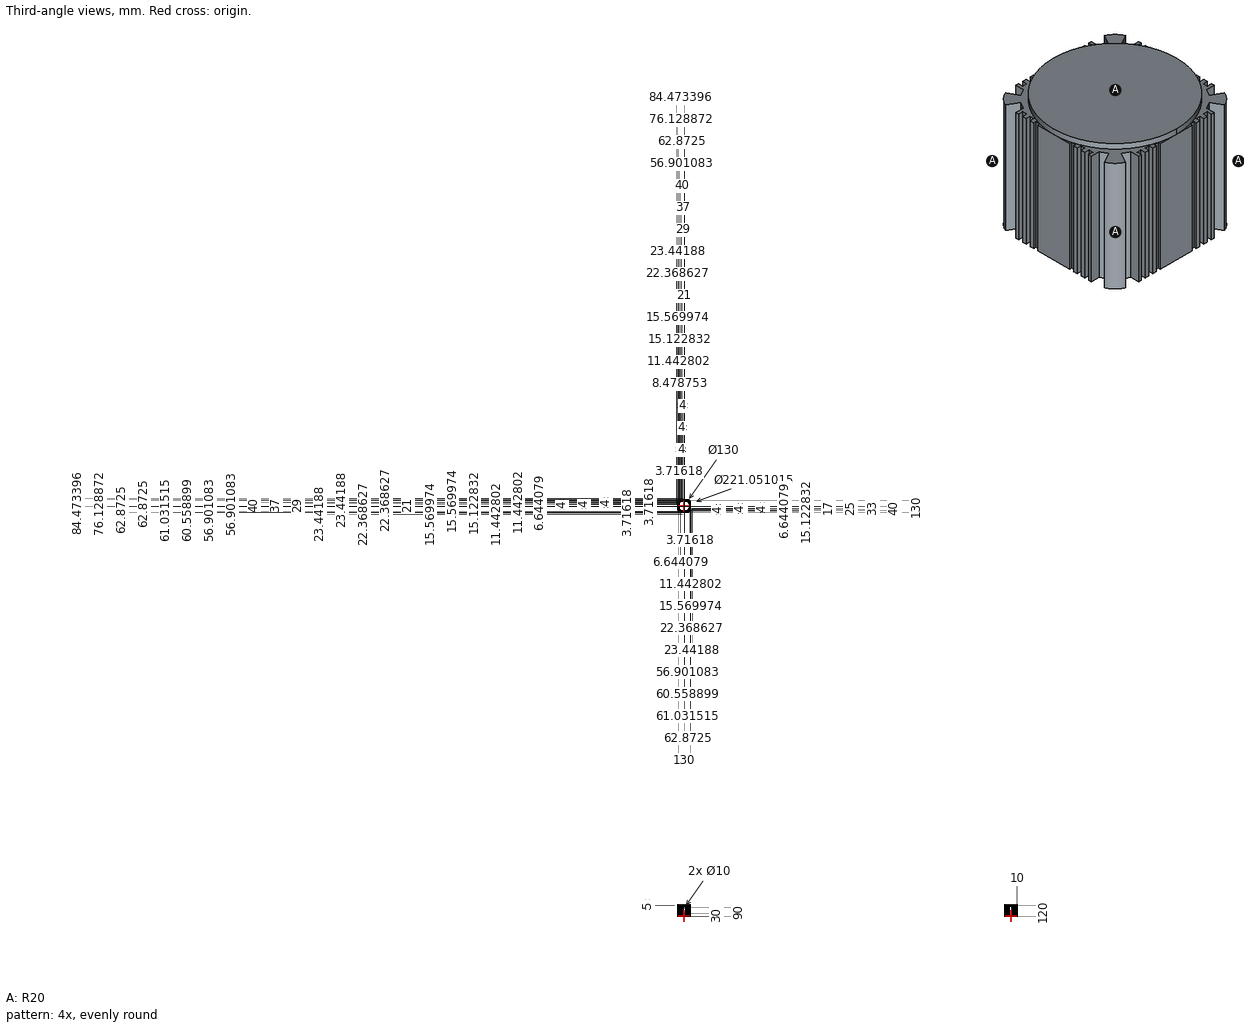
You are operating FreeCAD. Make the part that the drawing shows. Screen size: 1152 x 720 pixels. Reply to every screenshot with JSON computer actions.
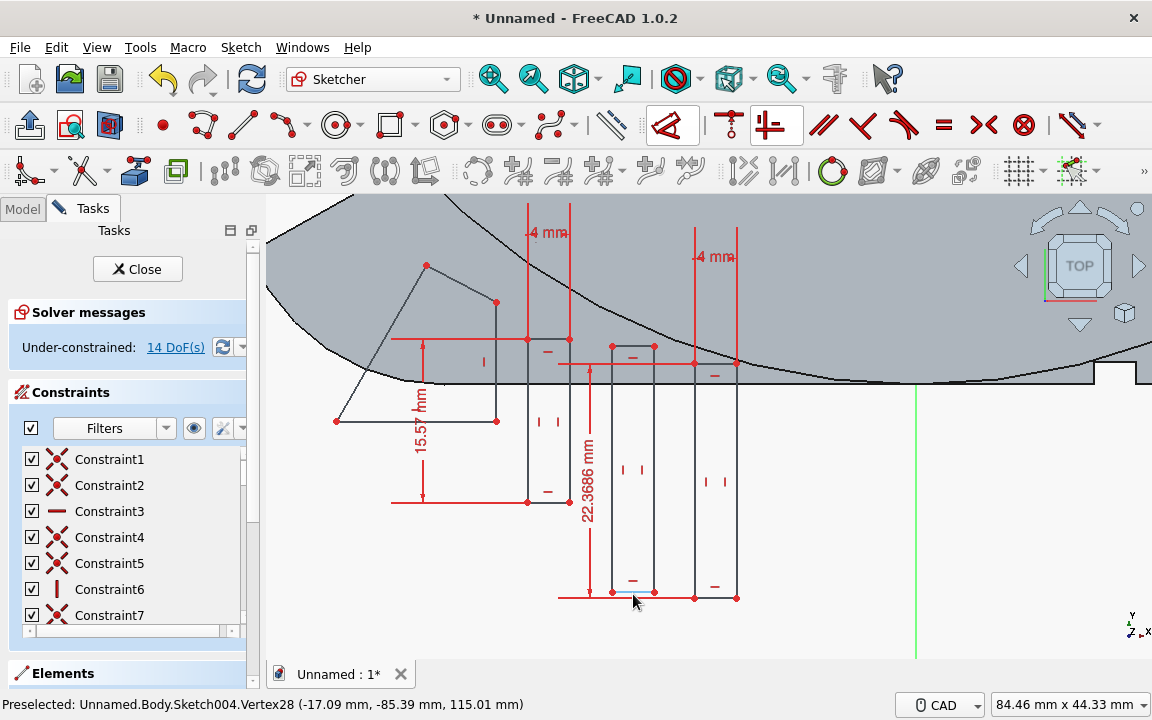
{"action": "left_click", "coordinate": [633, 592]}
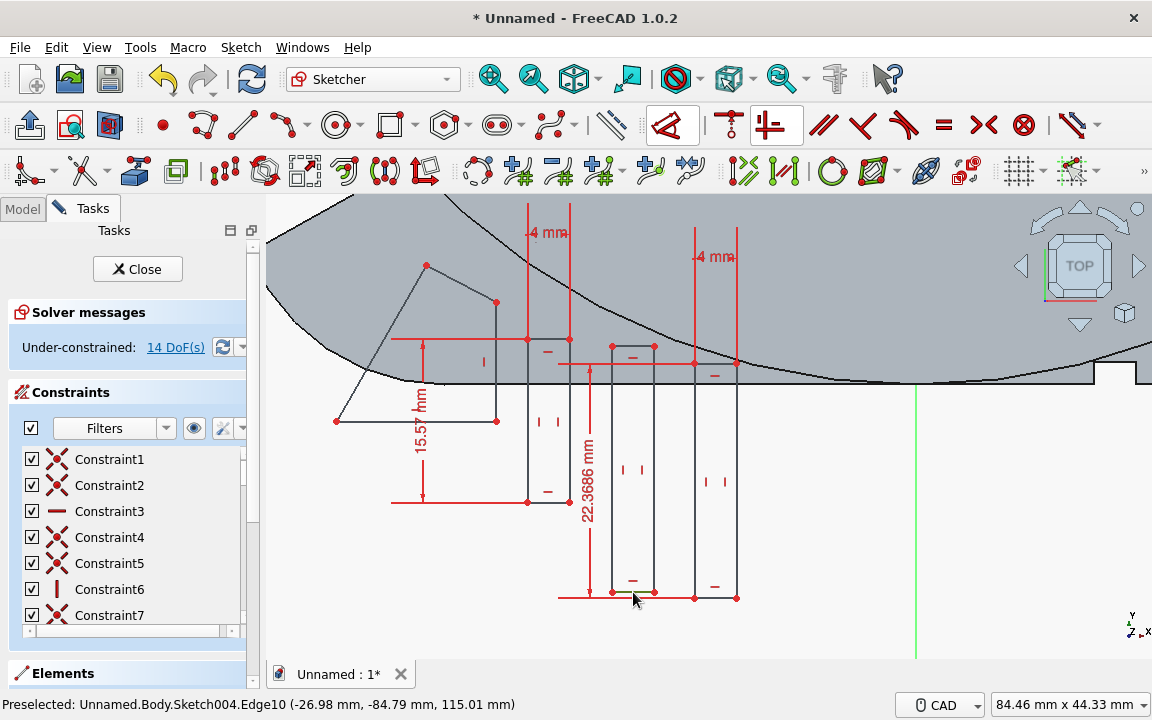
{"action": "key", "text": "l"}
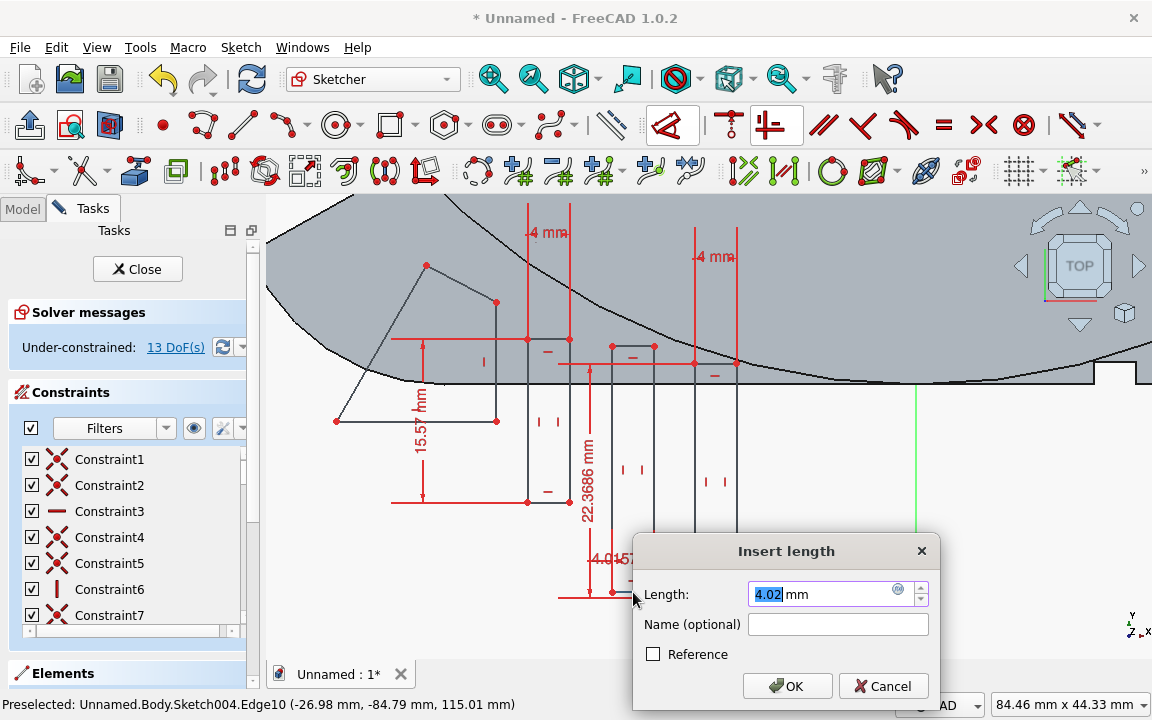
{"action": "type", "text": "4"}
{"action": "key", "text": "Return"}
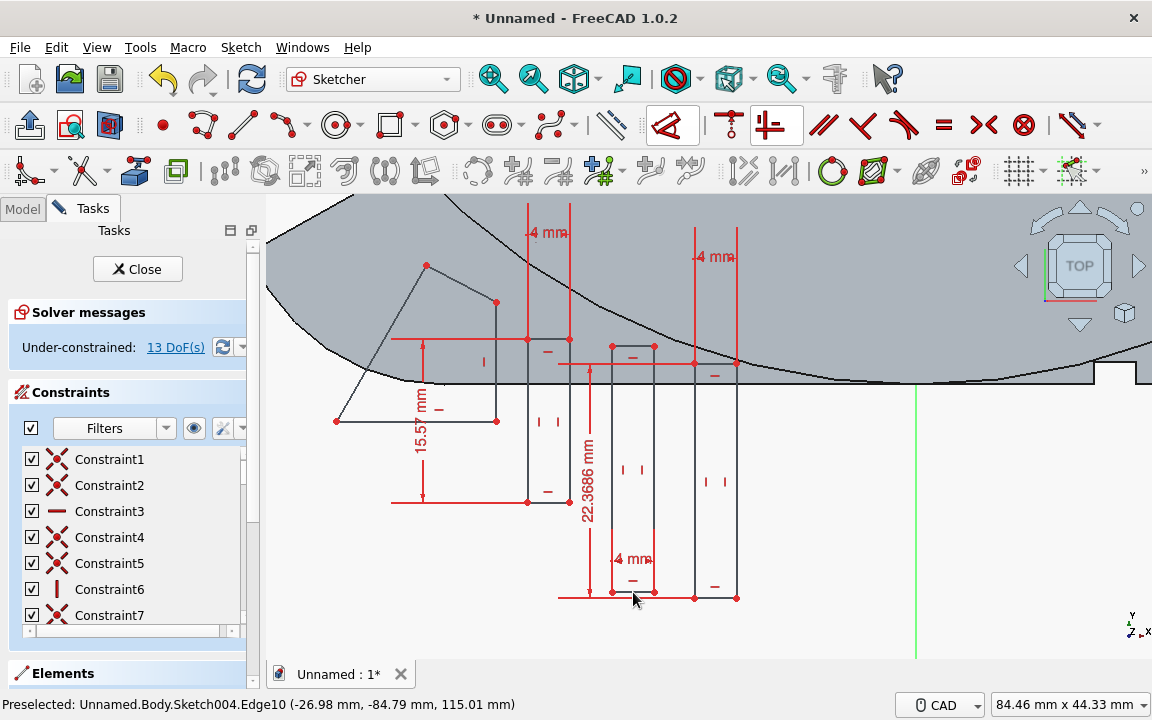
{"action": "left_click", "coordinate": [496, 302]}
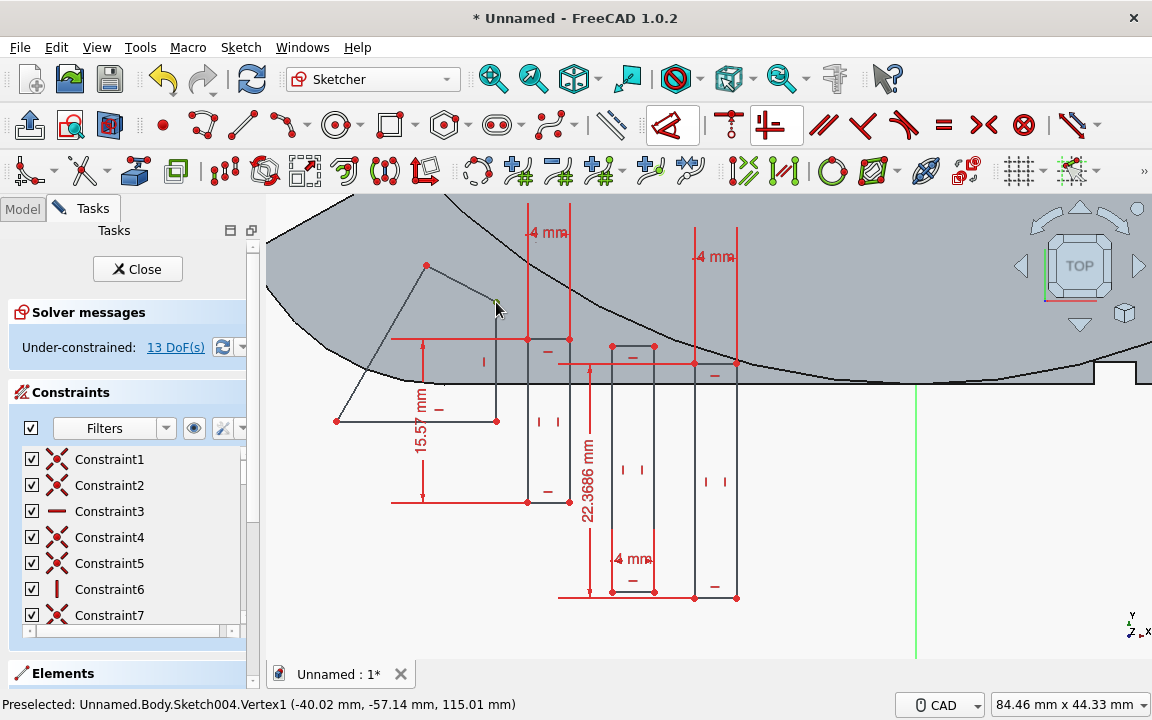
{"action": "key", "text": "l"}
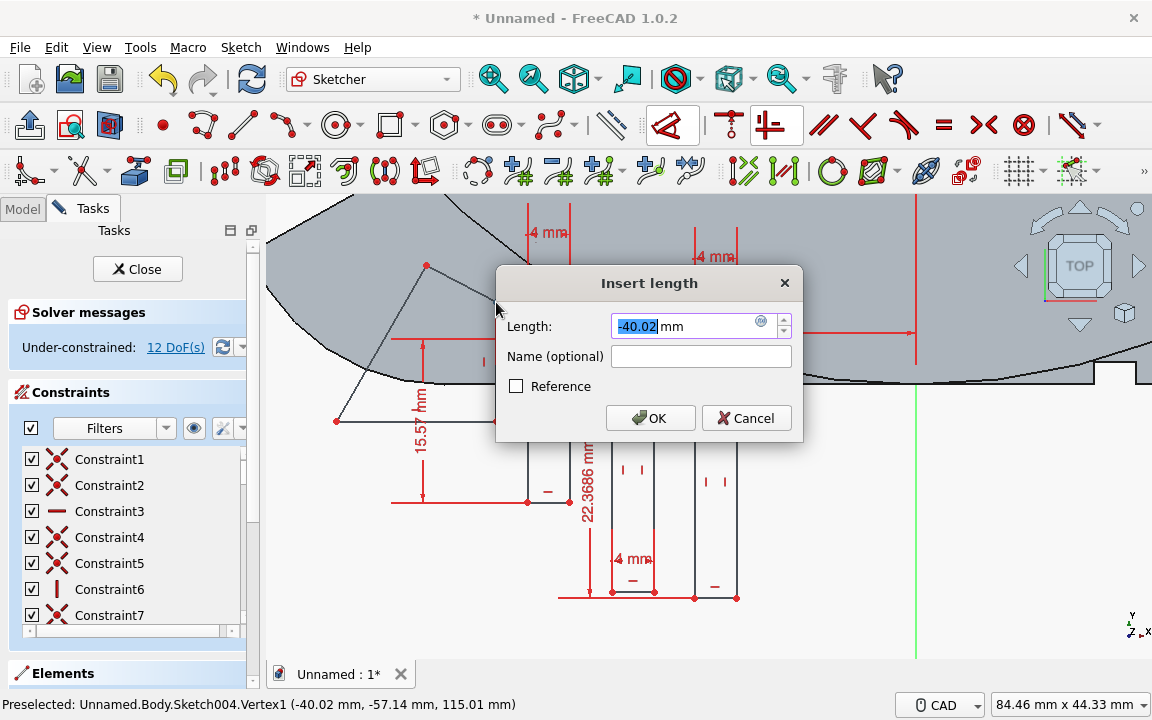
{"action": "type", "text": "-40"}
{"action": "key", "text": "Return"}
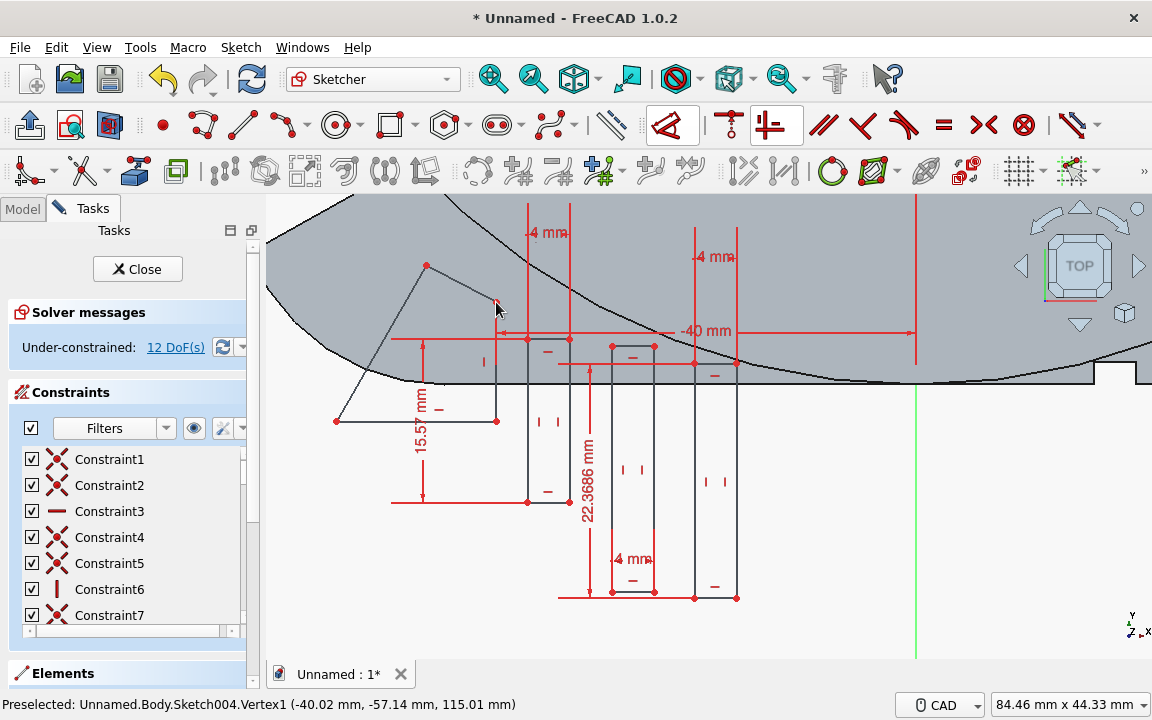
{"action": "left_click", "coordinate": [528, 339]}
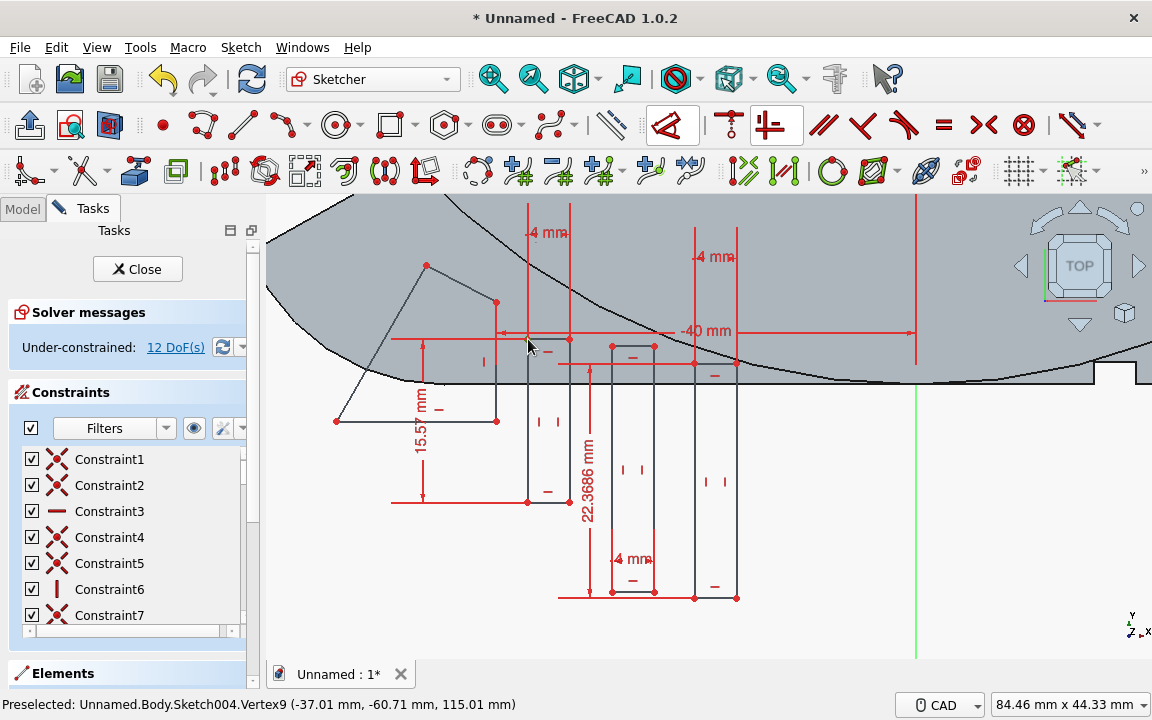
{"action": "key", "text": "l"}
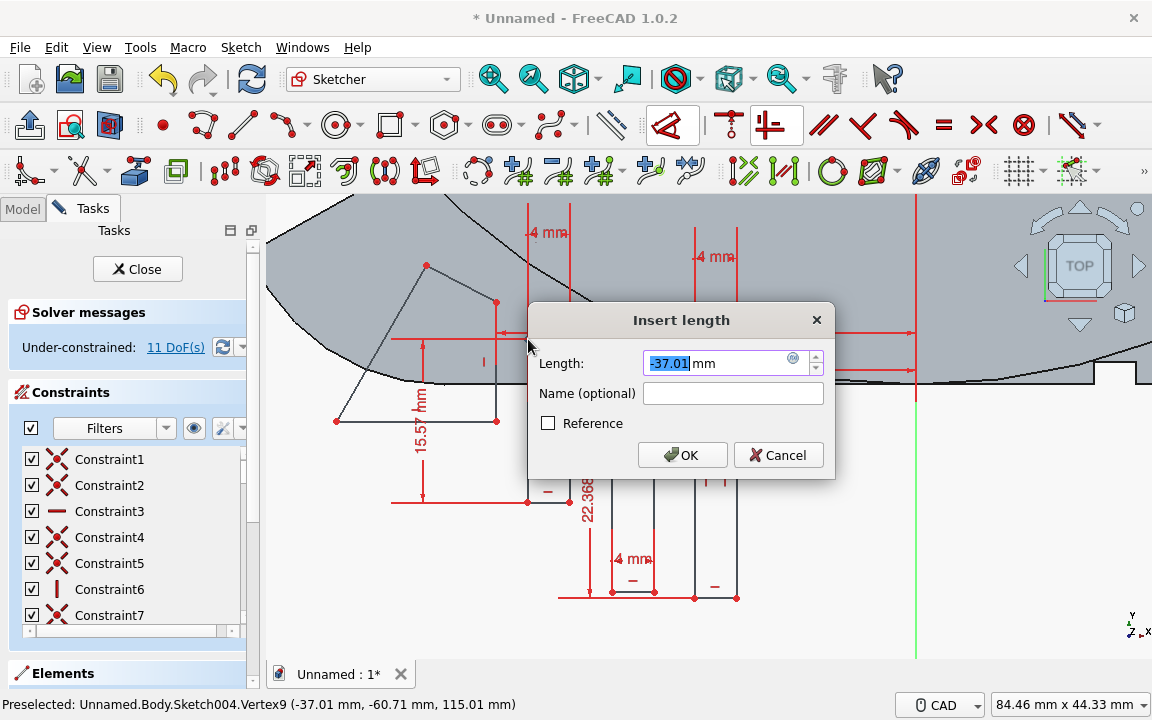
{"action": "type", "text": "-37"}
{"action": "key", "text": "Return"}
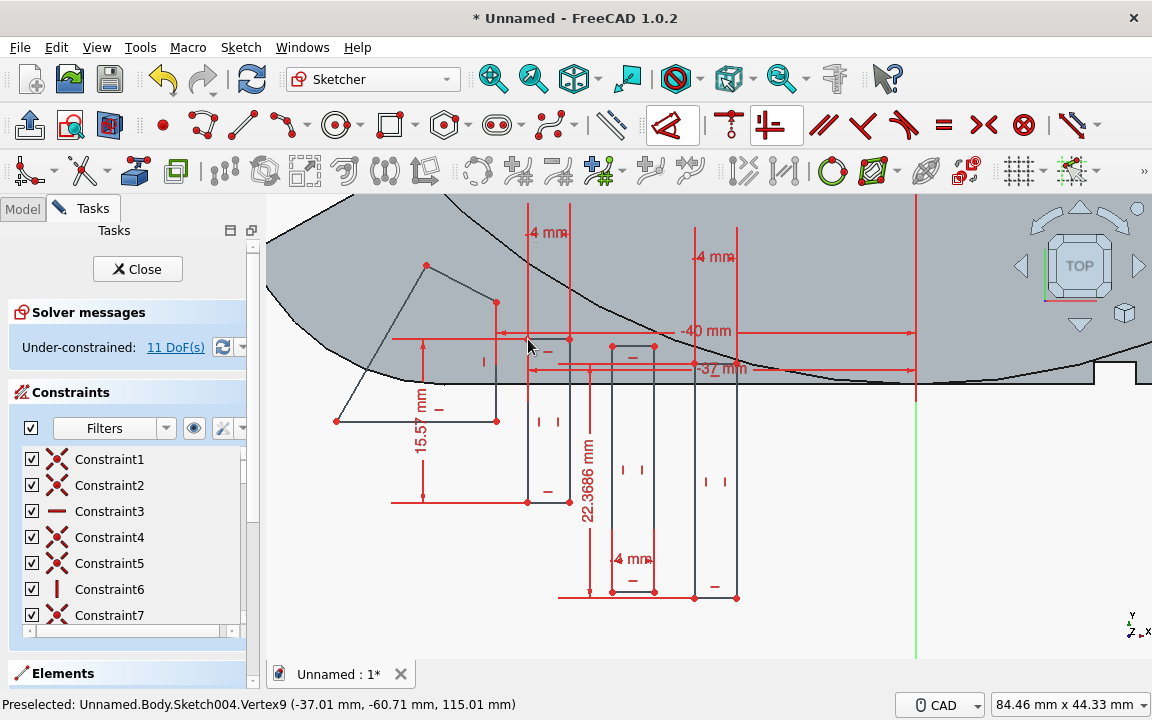
{"action": "left_click", "coordinate": [612, 346]}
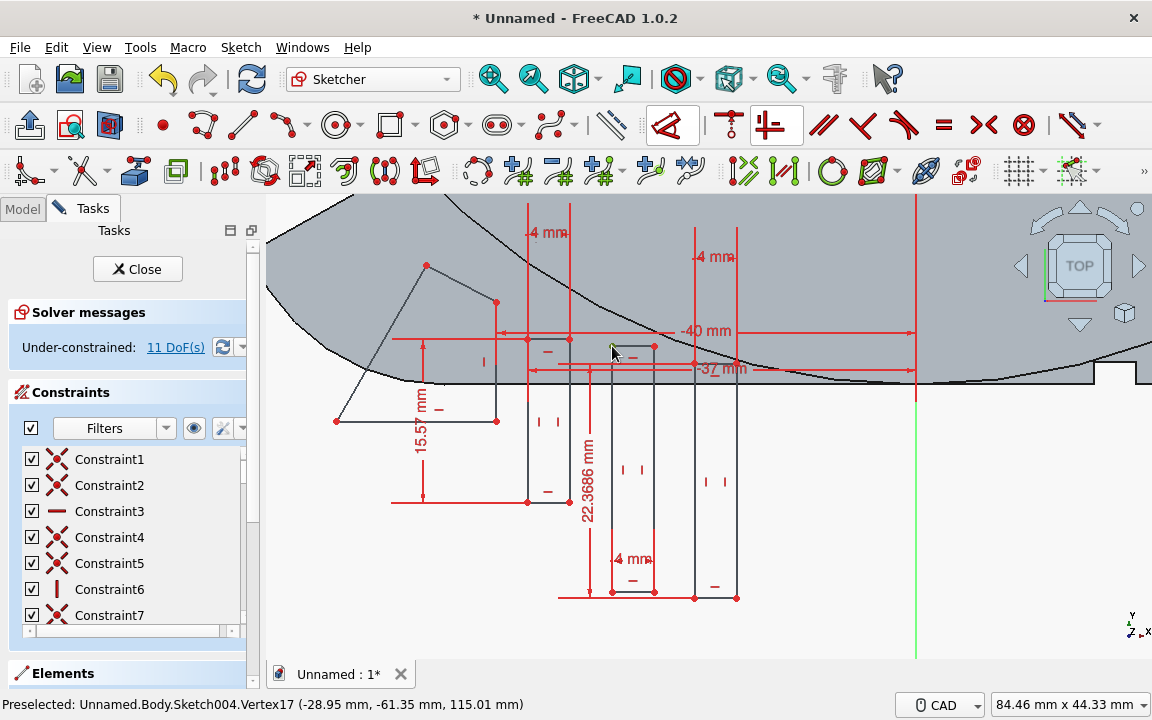
{"action": "key", "text": "l"}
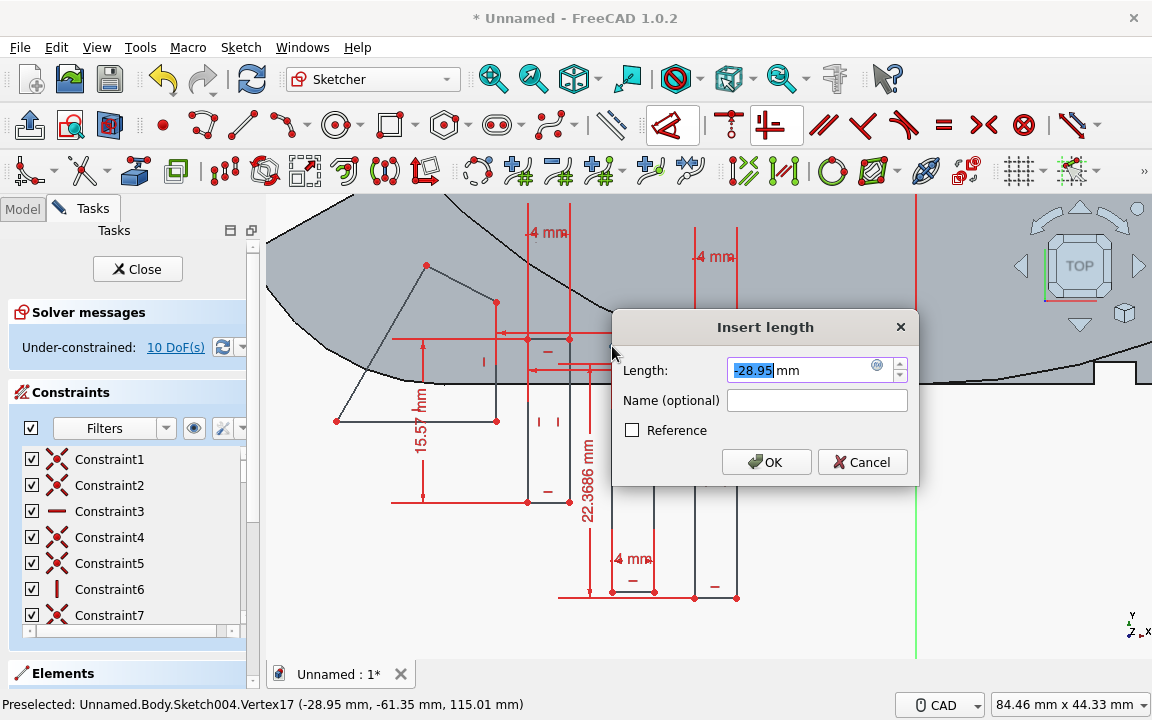
{"action": "type", "text": "-29"}
{"action": "key", "text": "Return"}